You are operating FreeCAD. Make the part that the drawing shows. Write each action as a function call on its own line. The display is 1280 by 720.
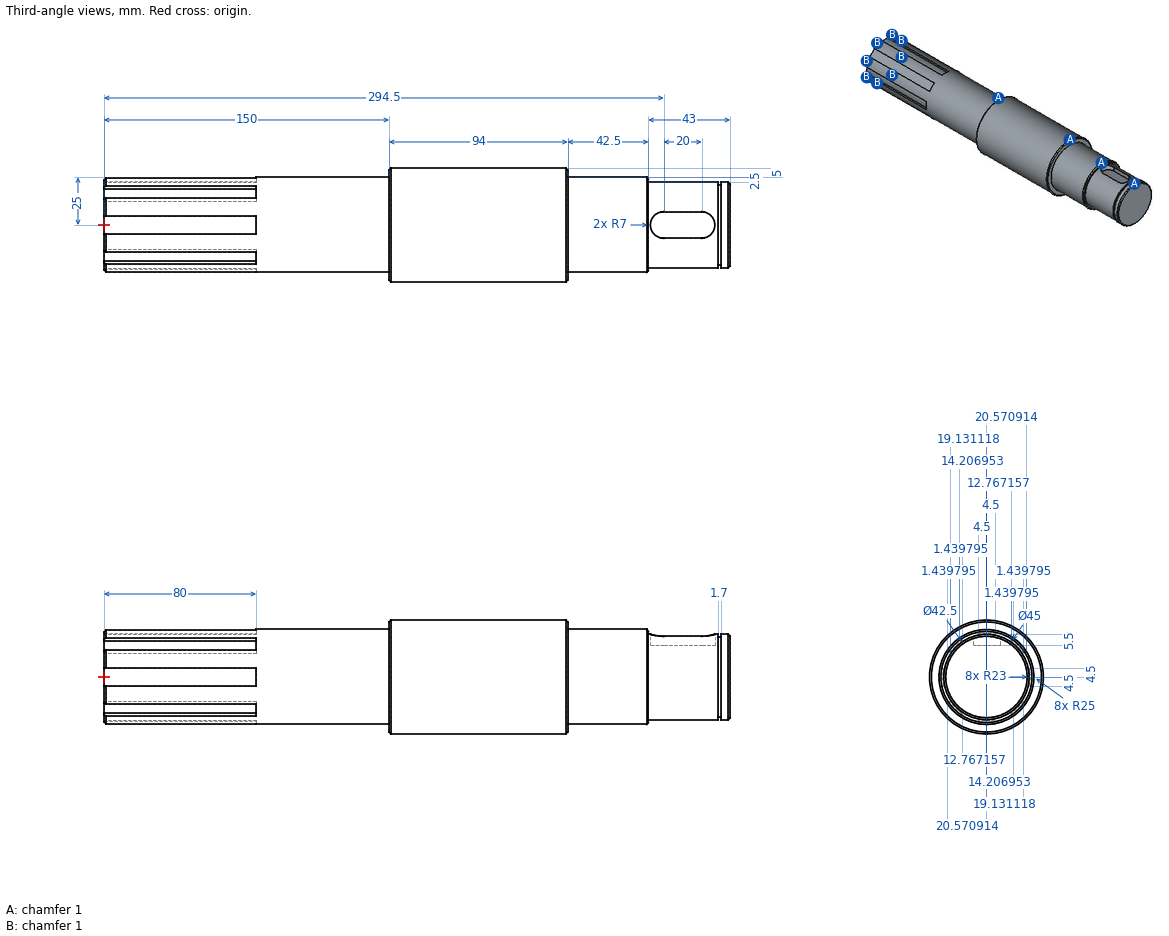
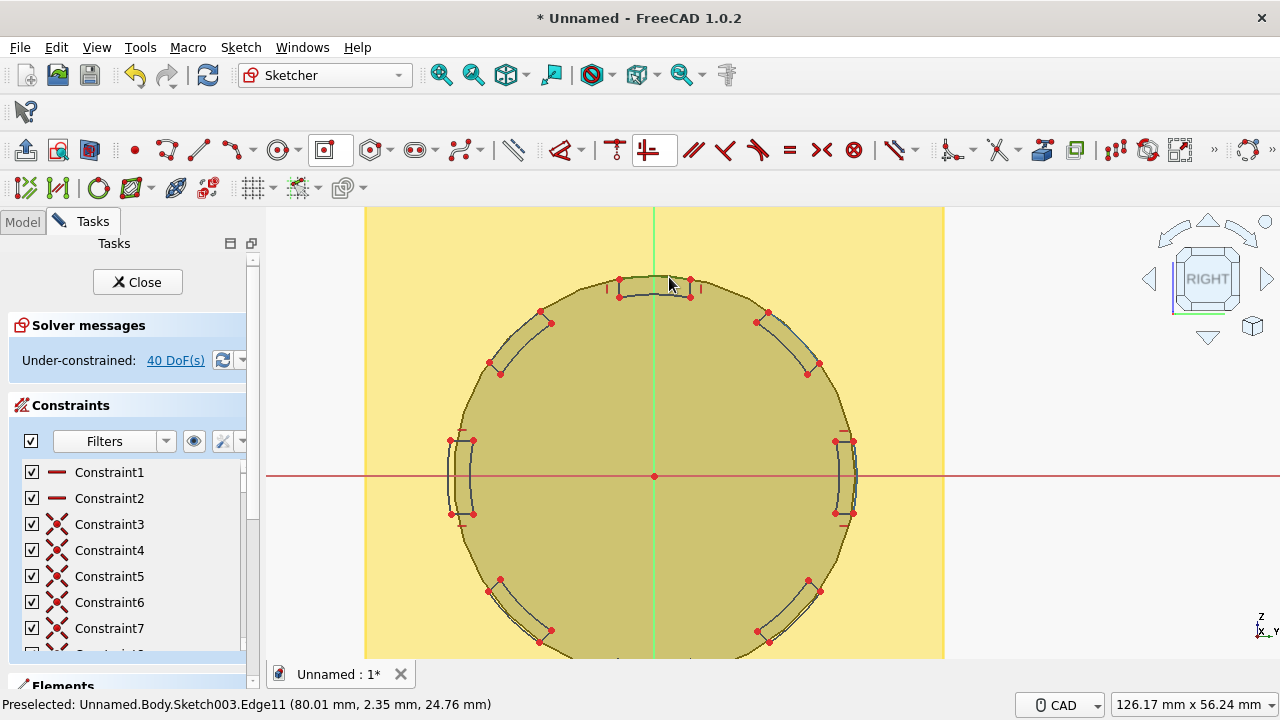
click(524, 325)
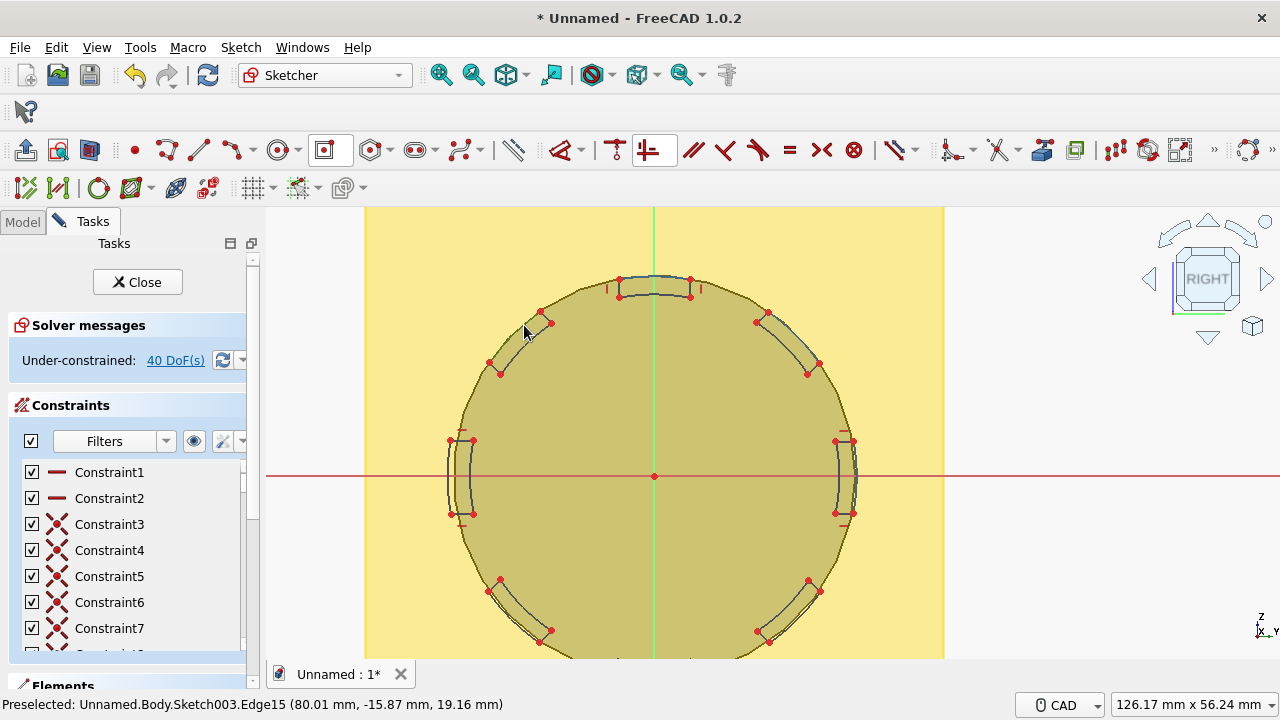
click(448, 463)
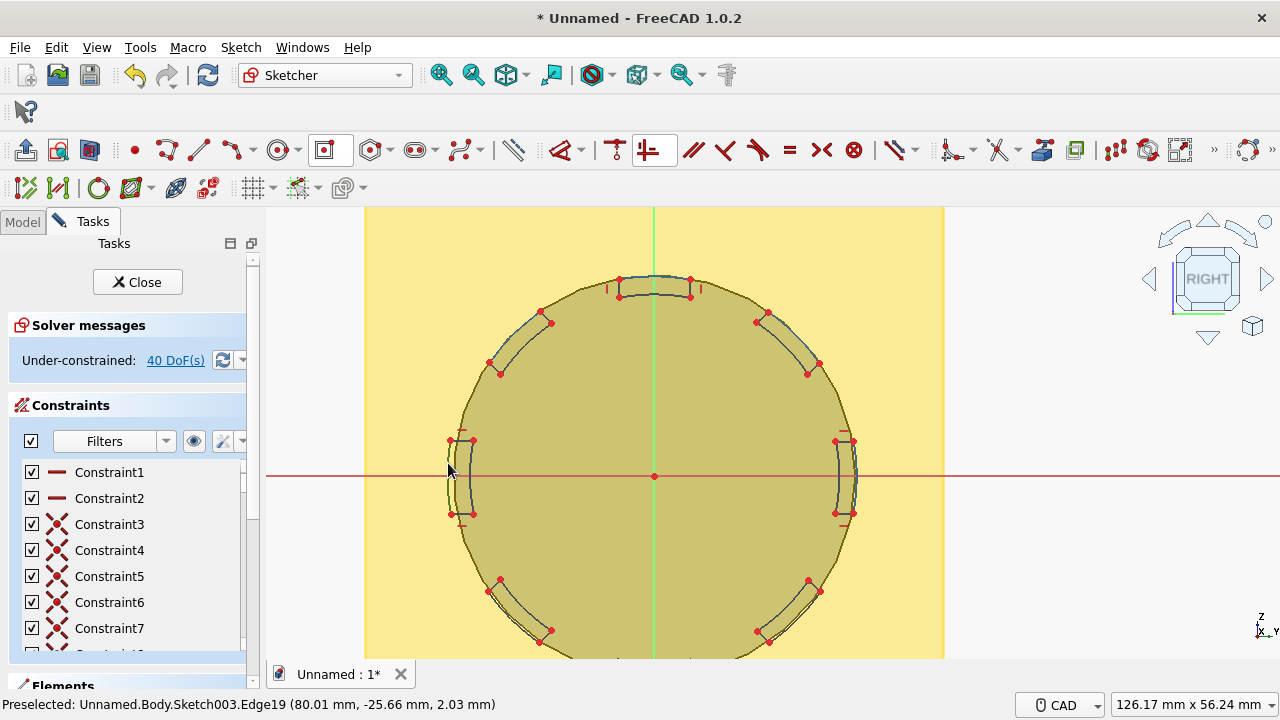
click(502, 609)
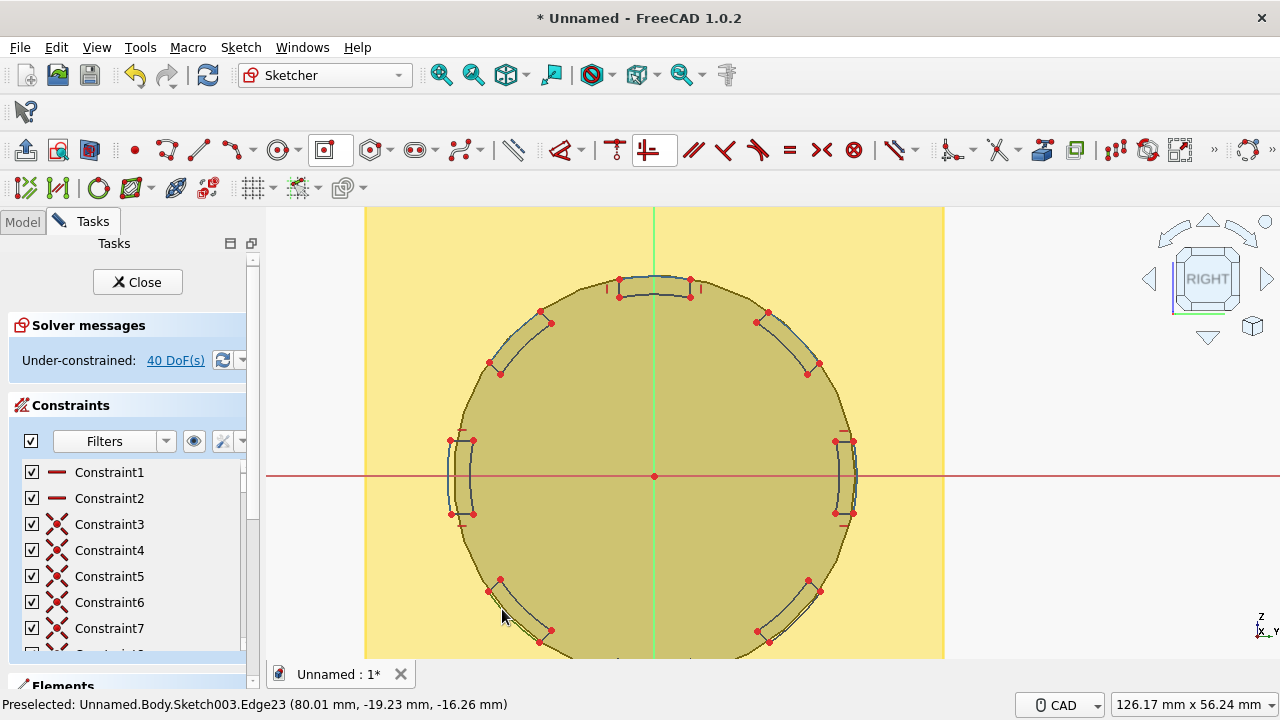
scroll(806, 345, down, 2)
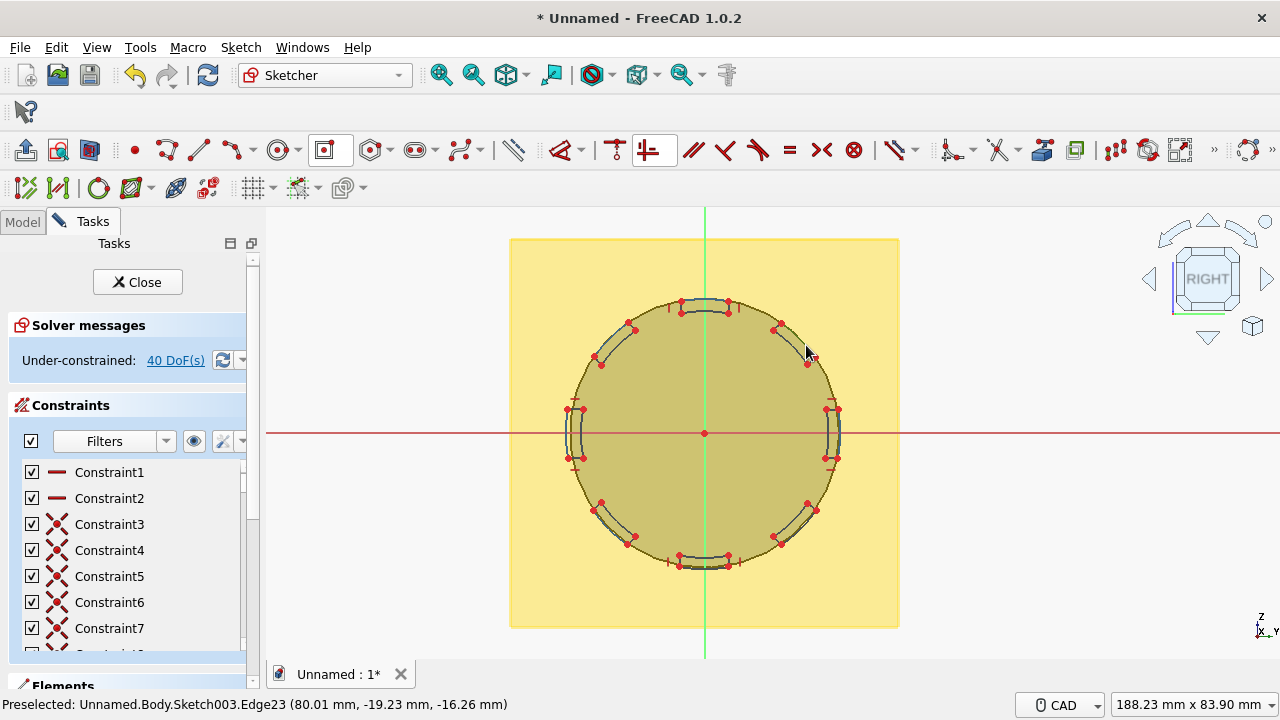
scroll(695, 569, up, 2)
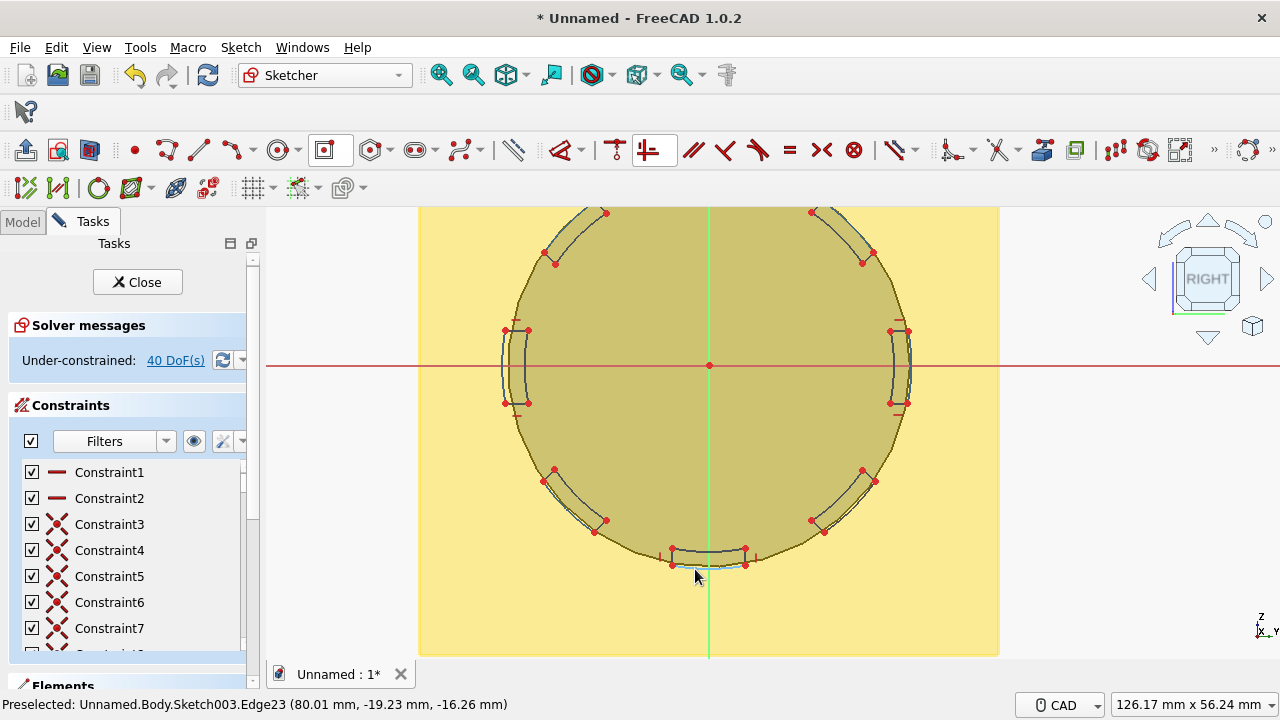
click(694, 568)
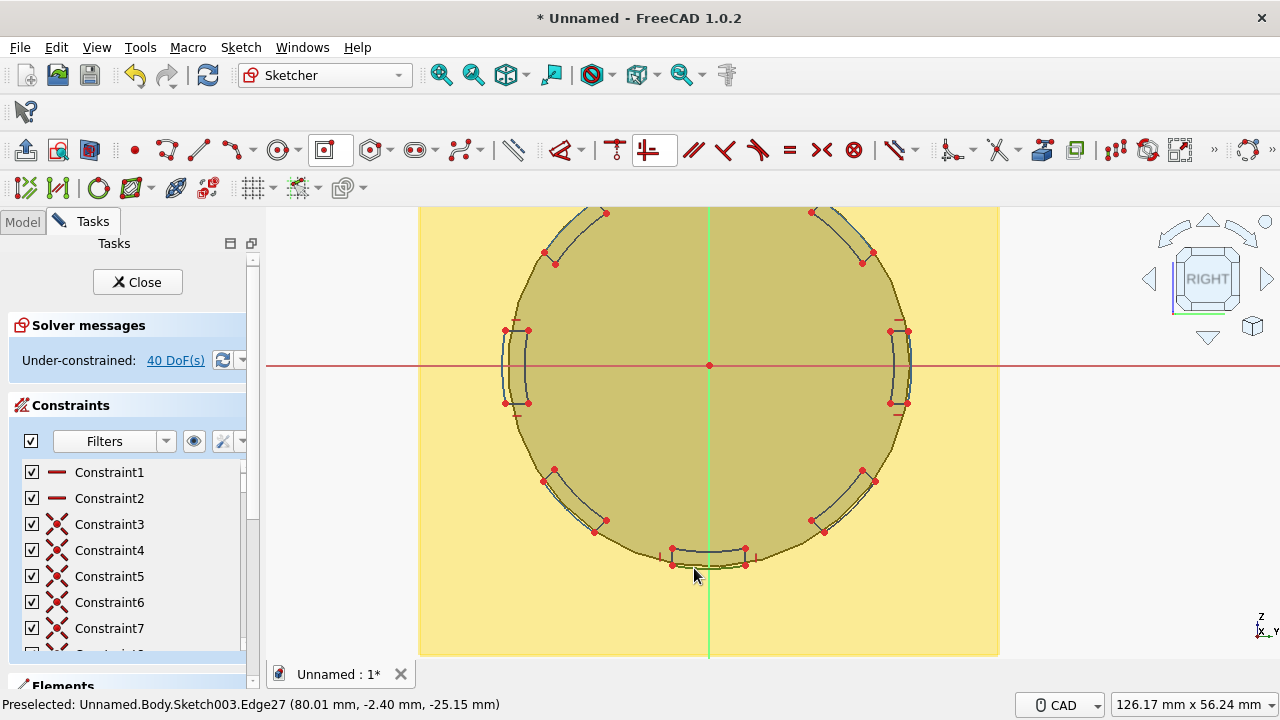
click(841, 519)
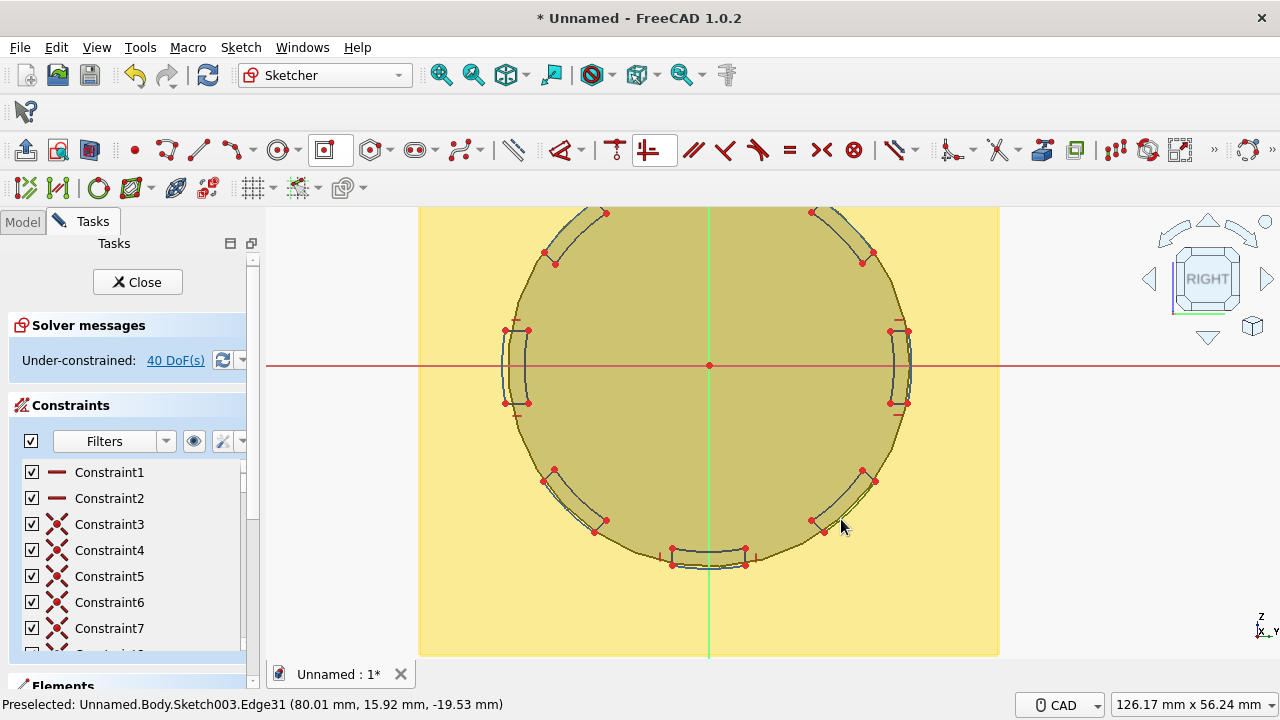
click(790, 150)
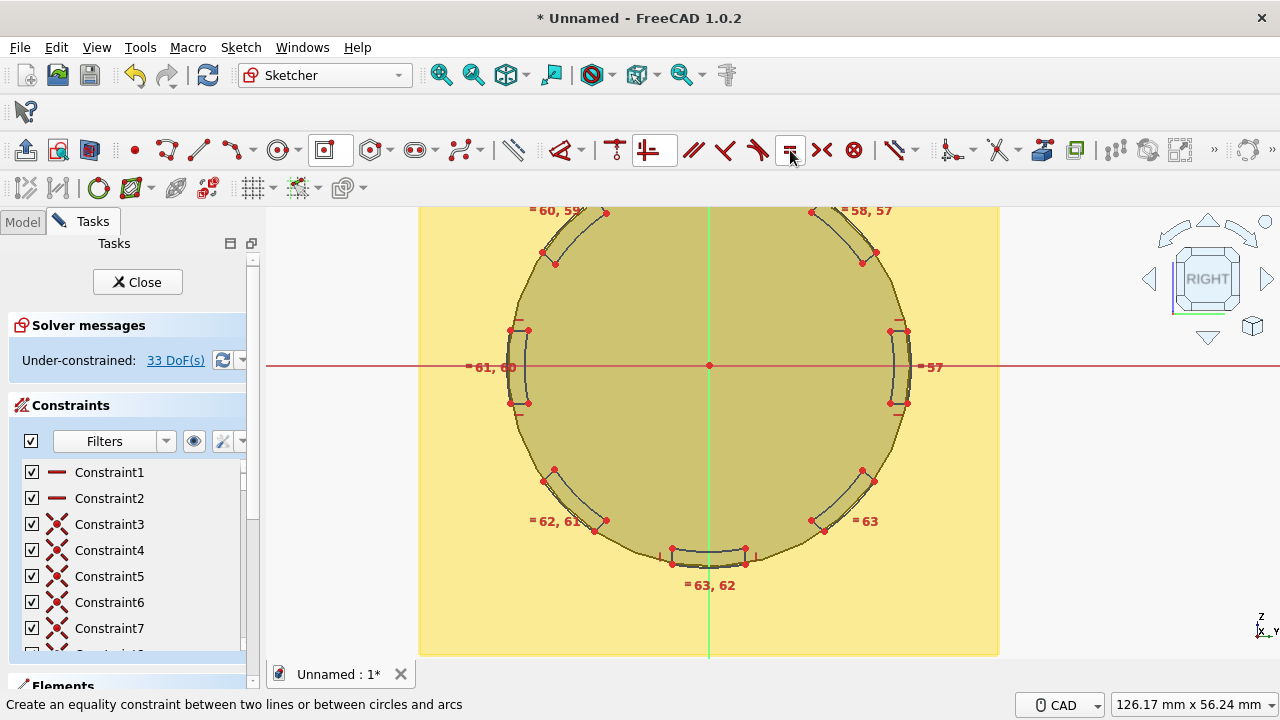
click(893, 382)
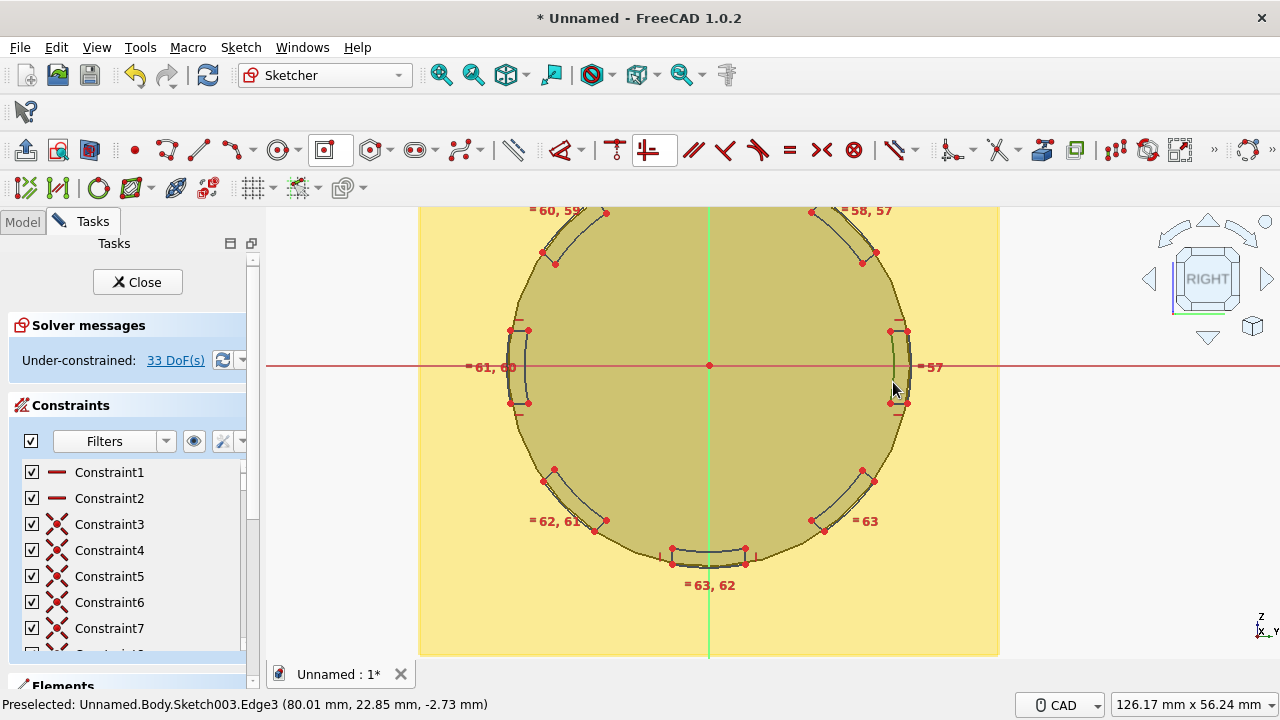
click(849, 246)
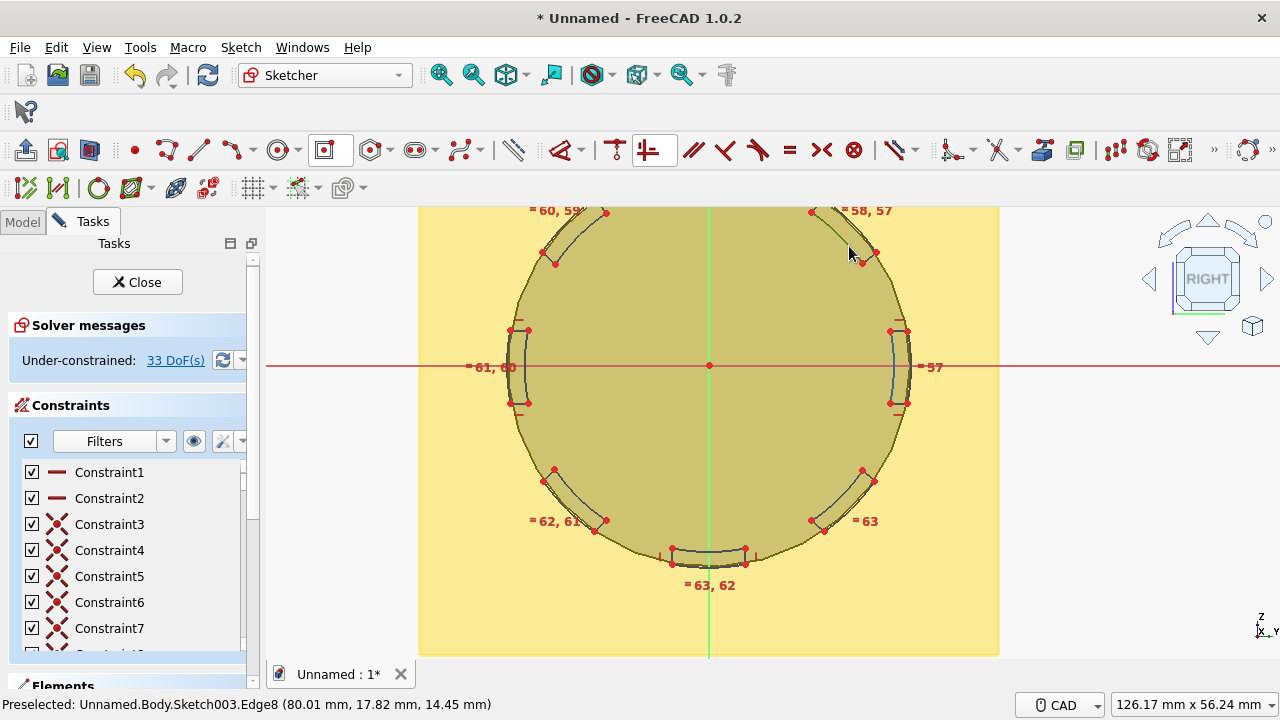
scroll(695, 570, down, 2)